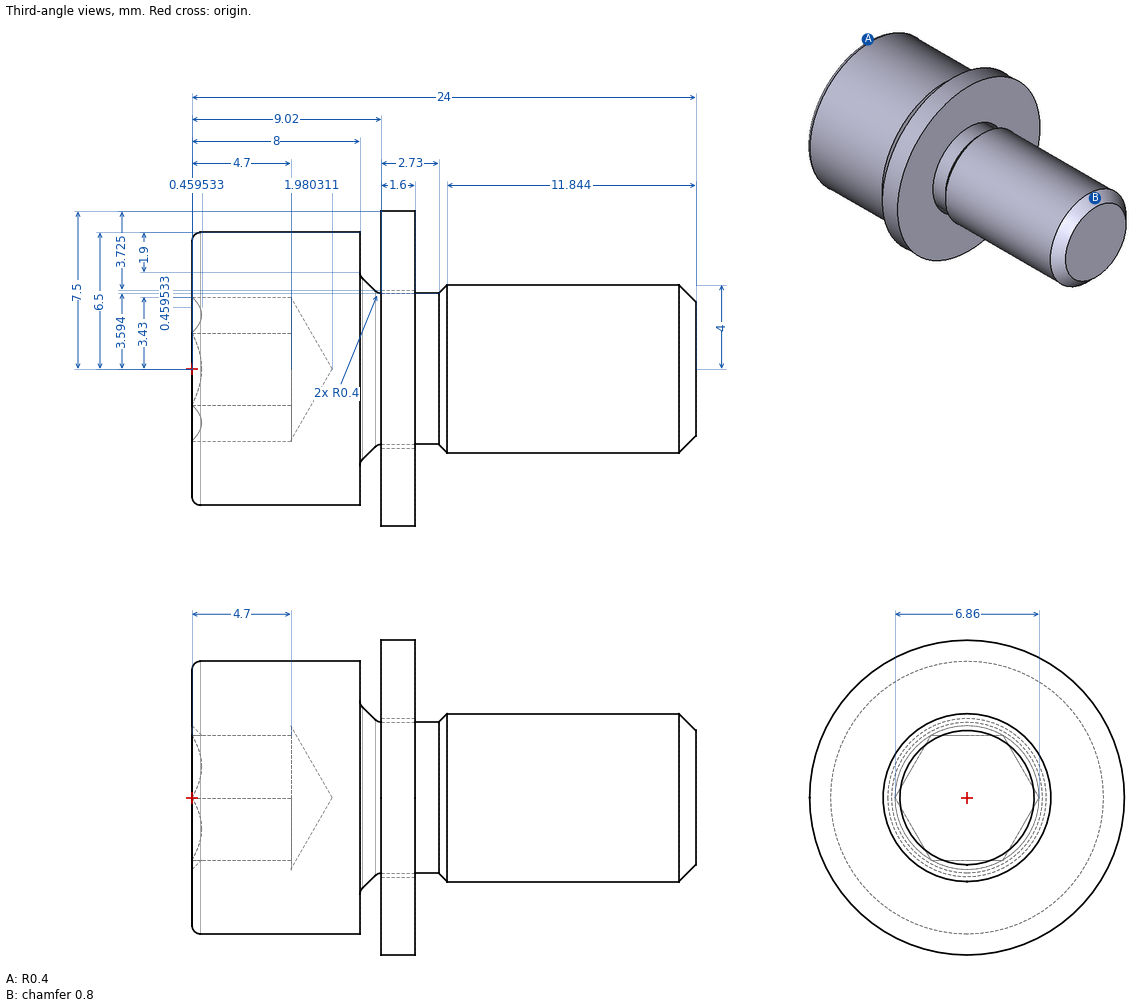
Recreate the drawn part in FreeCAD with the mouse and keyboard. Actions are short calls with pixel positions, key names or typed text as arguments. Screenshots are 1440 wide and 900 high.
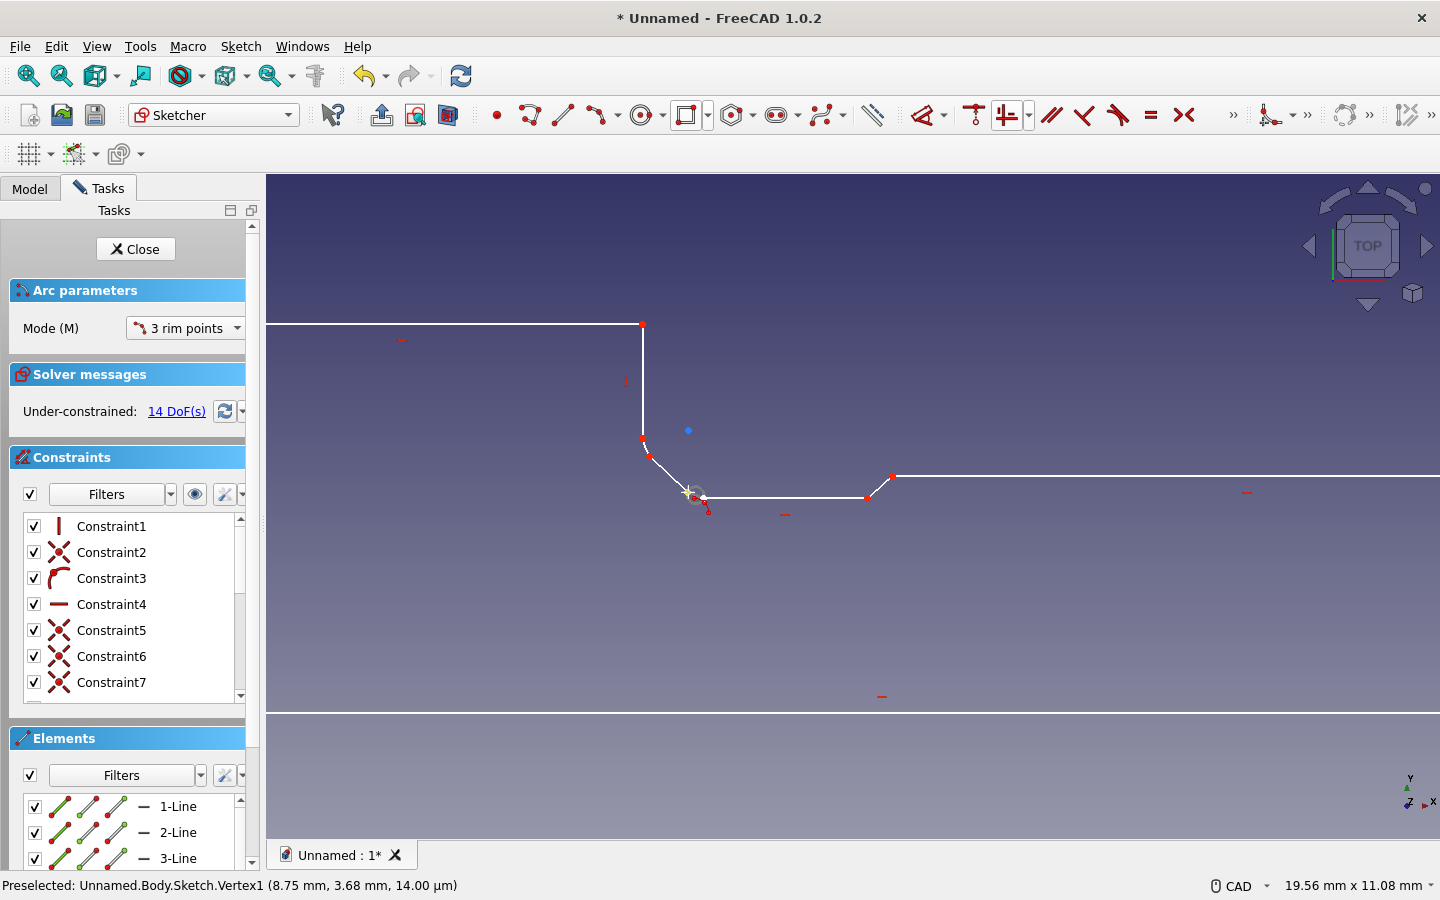
scroll(695, 495, up, 11)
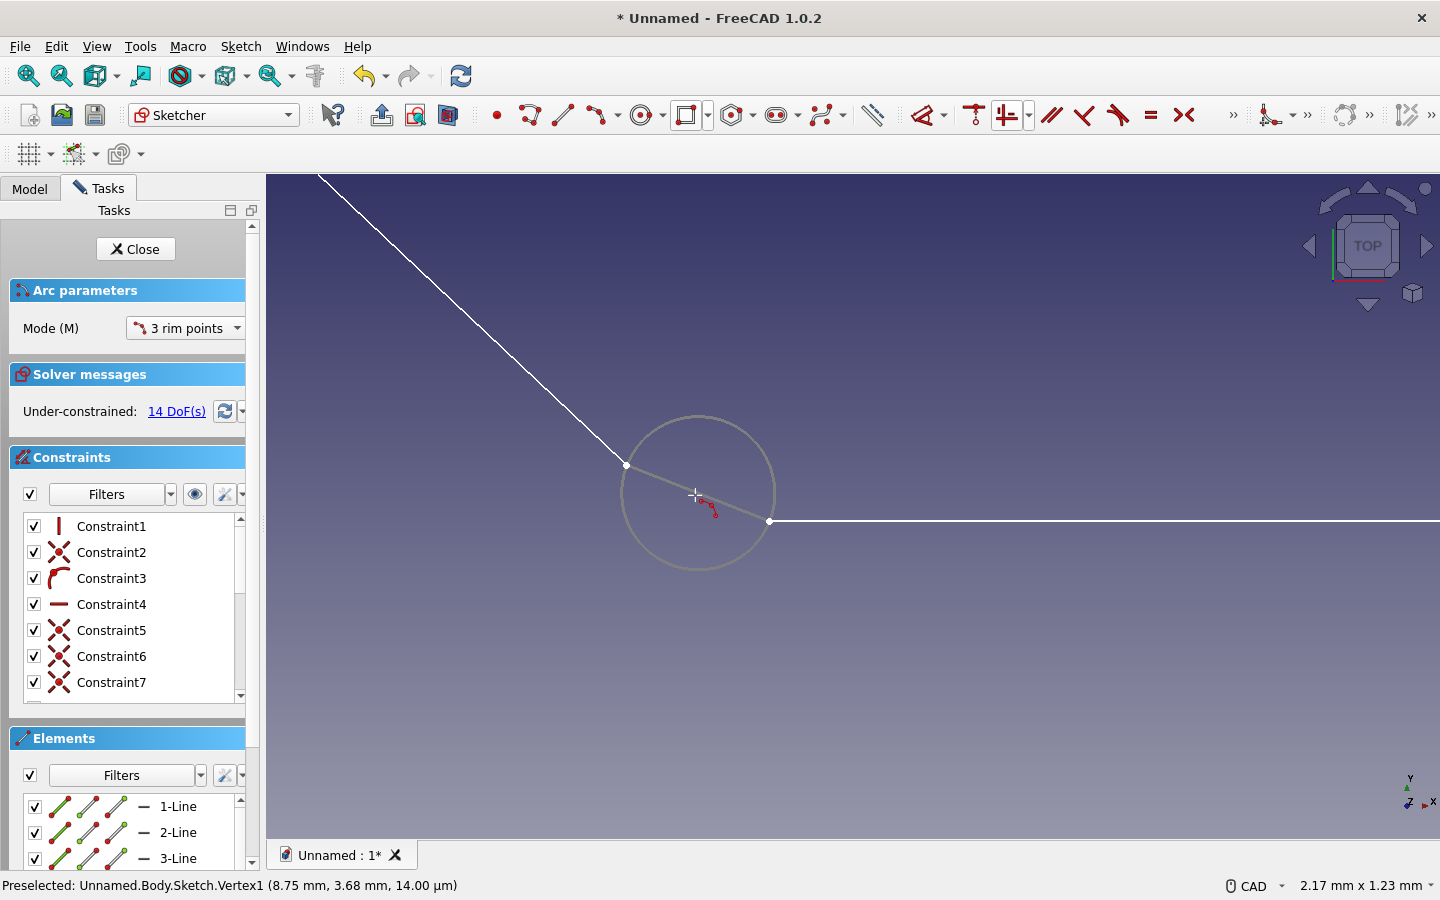
click(692, 494)
key(Escape)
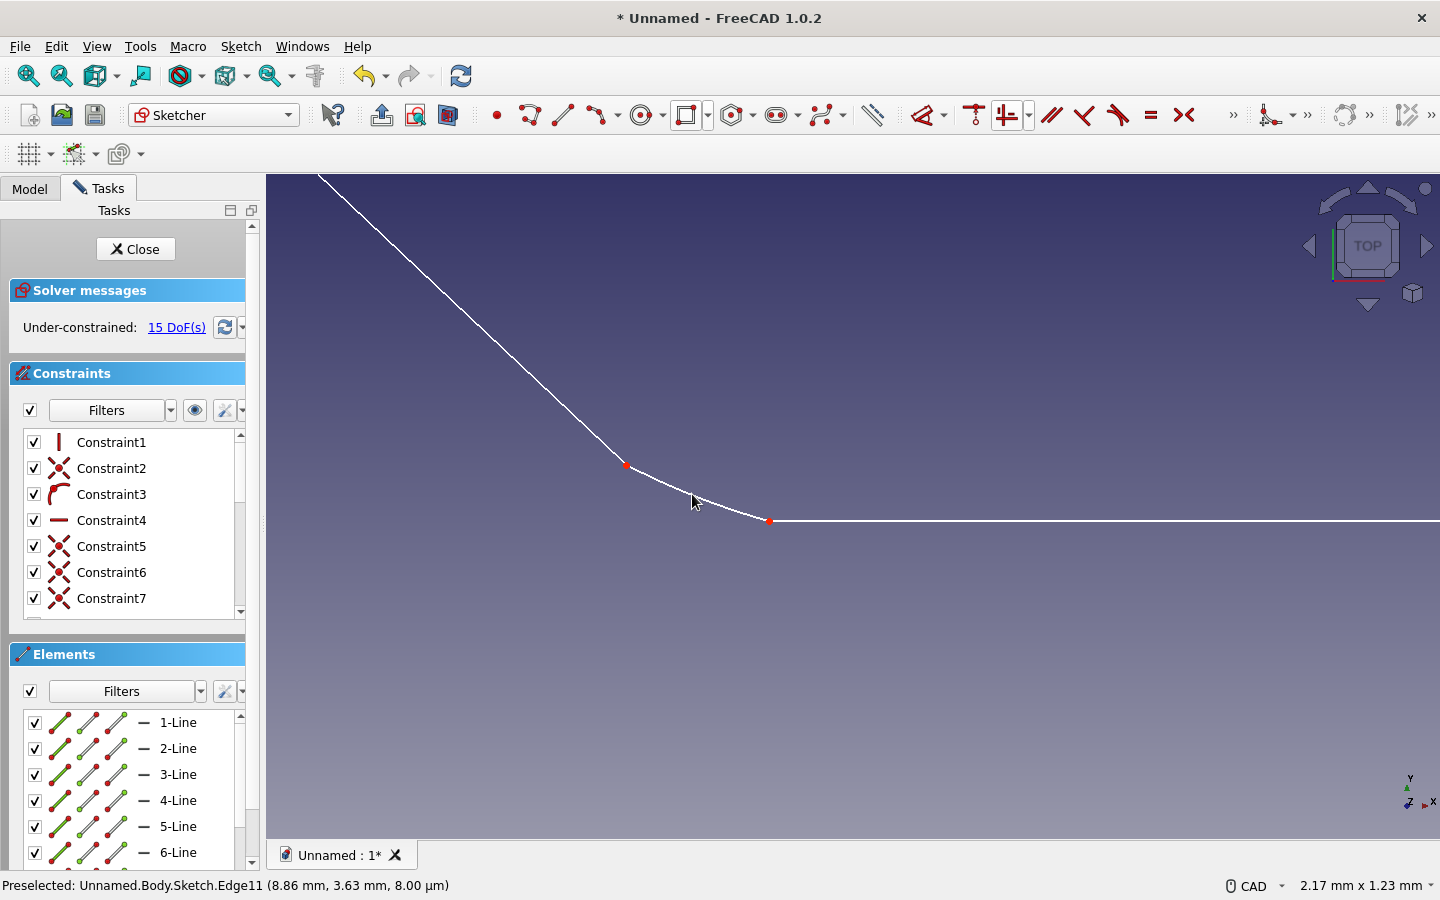
scroll(700, 497, down, 15)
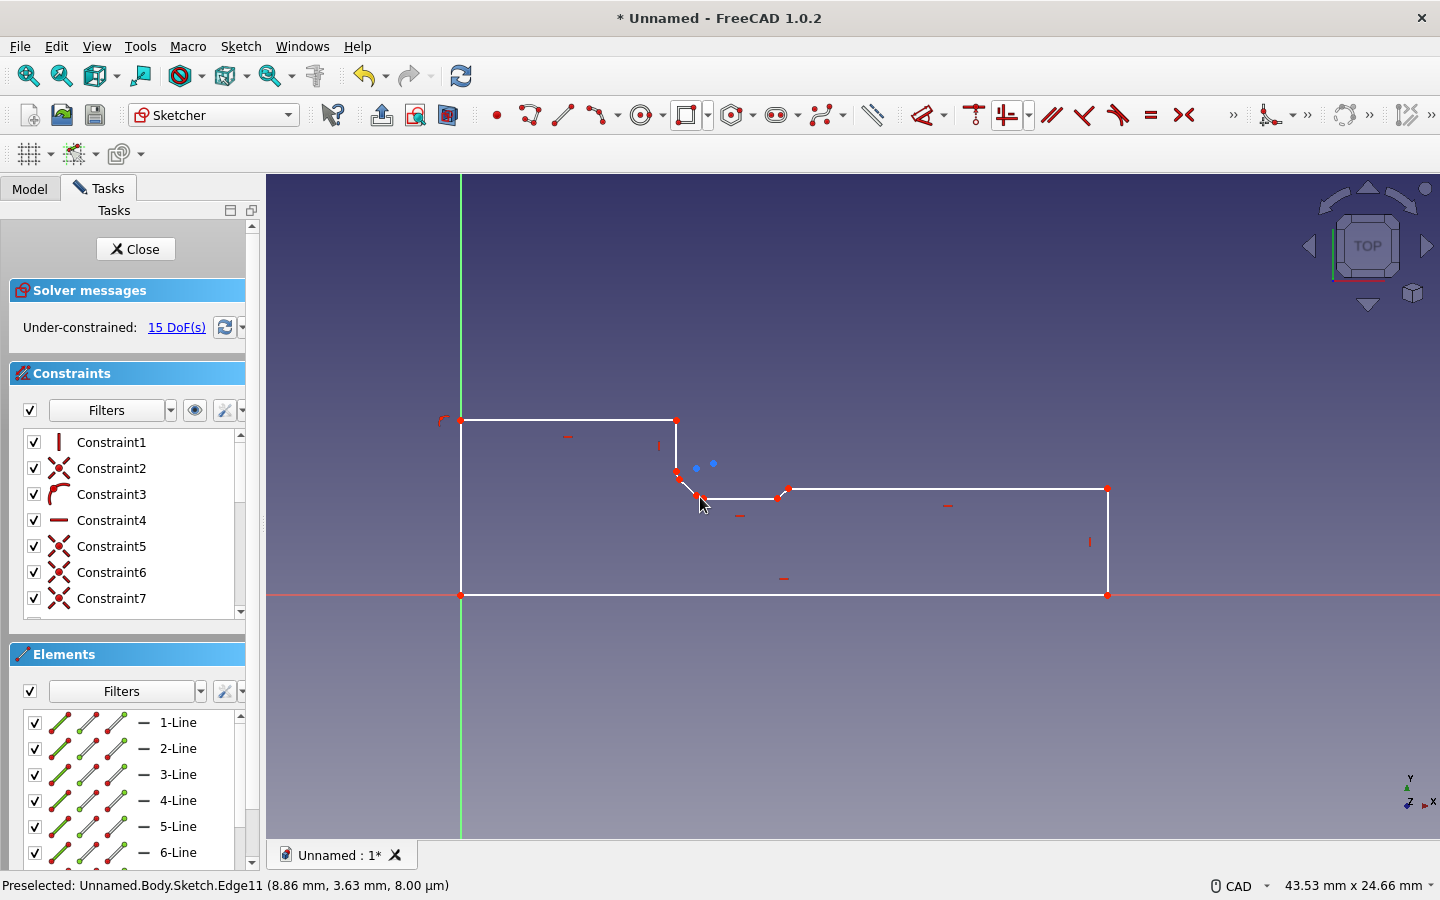
scroll(692, 491, up, 4)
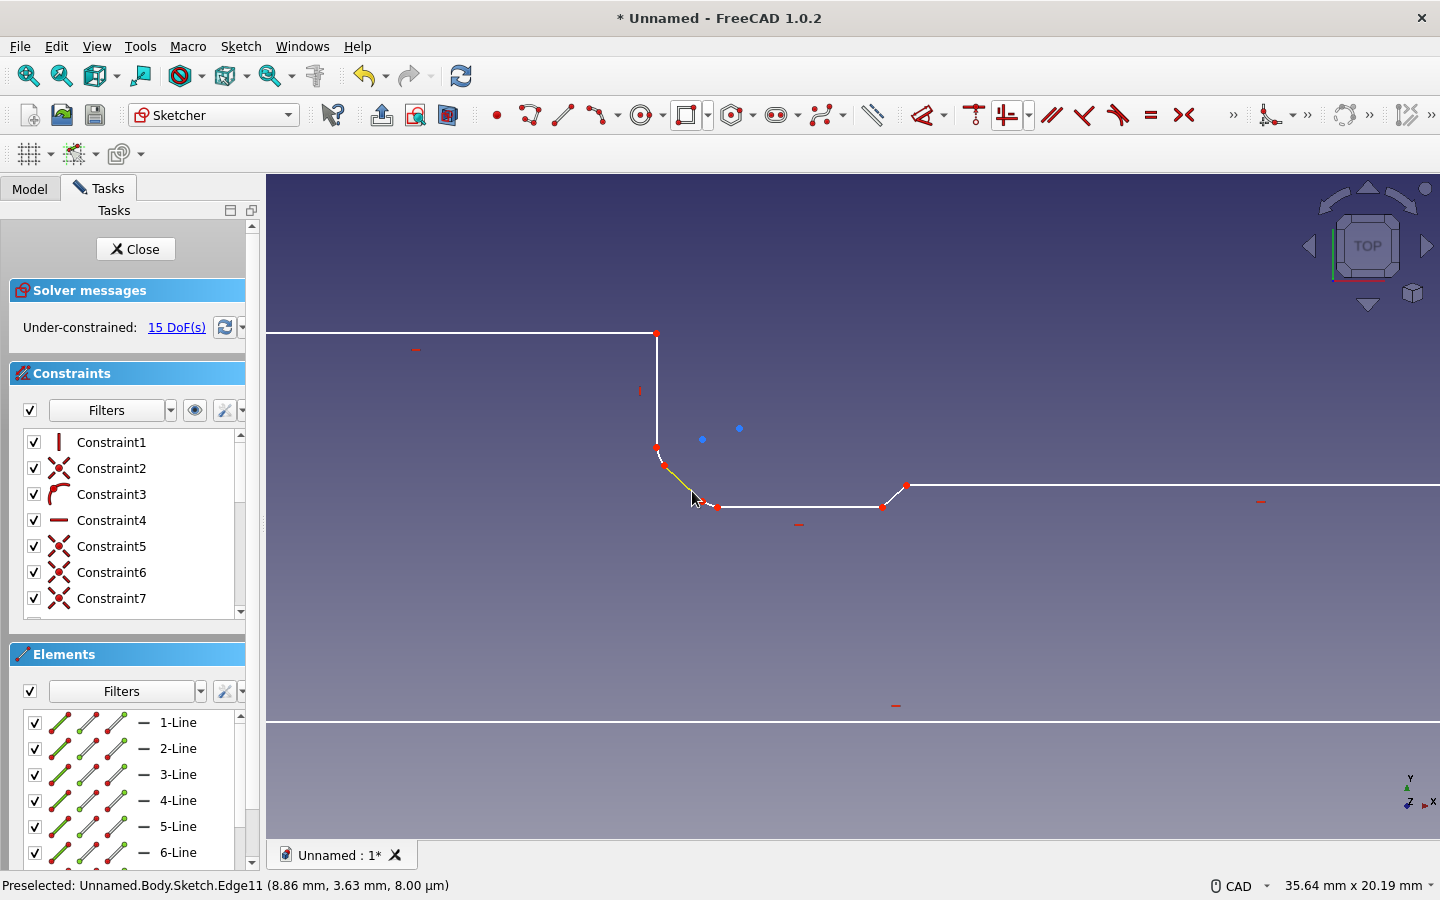
click(691, 491)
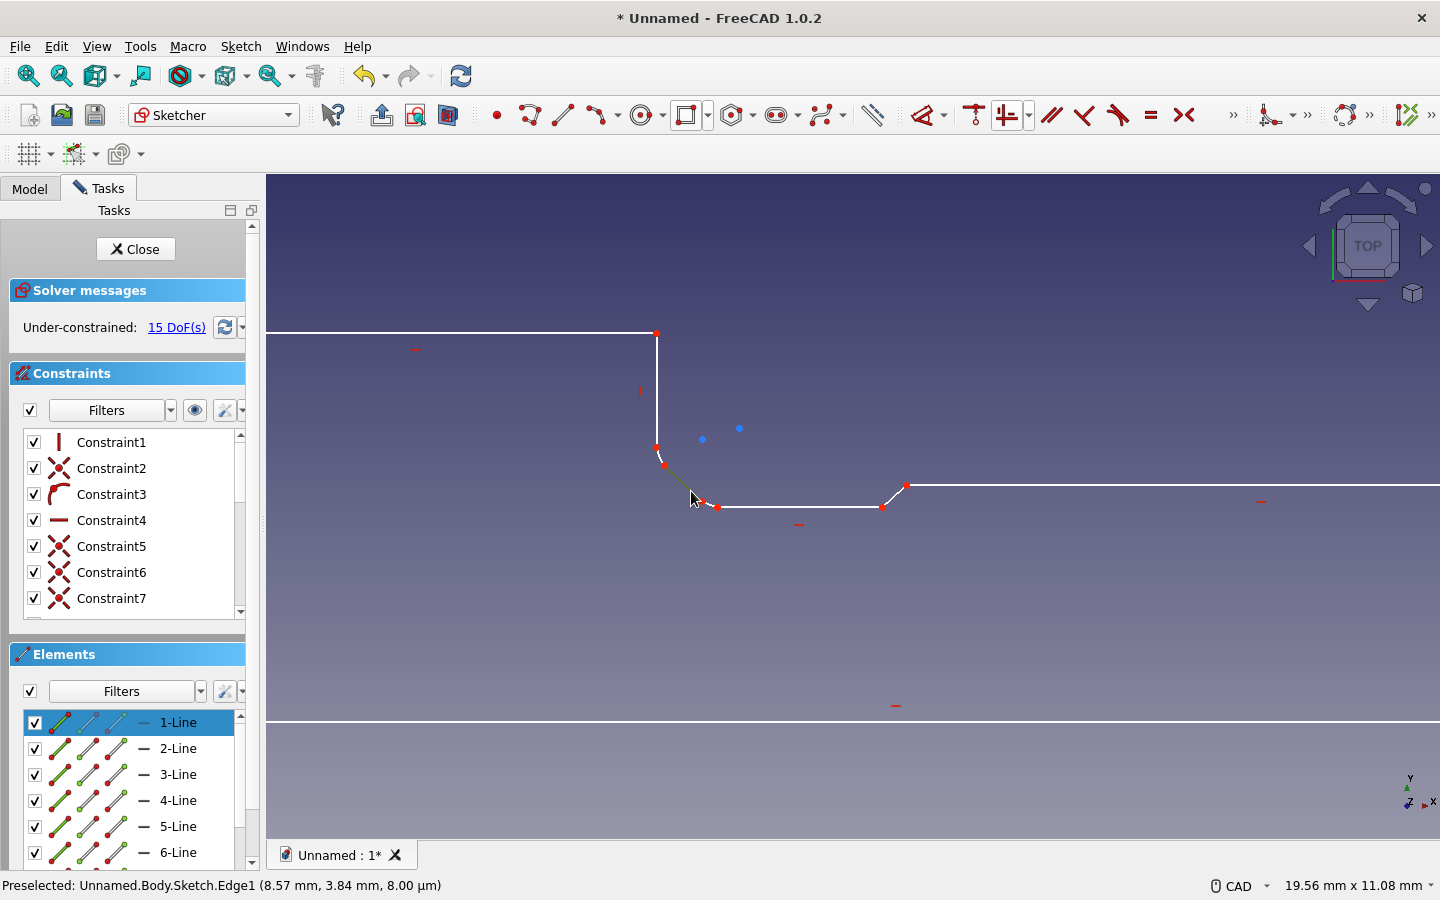
scroll(660, 457, up, 2)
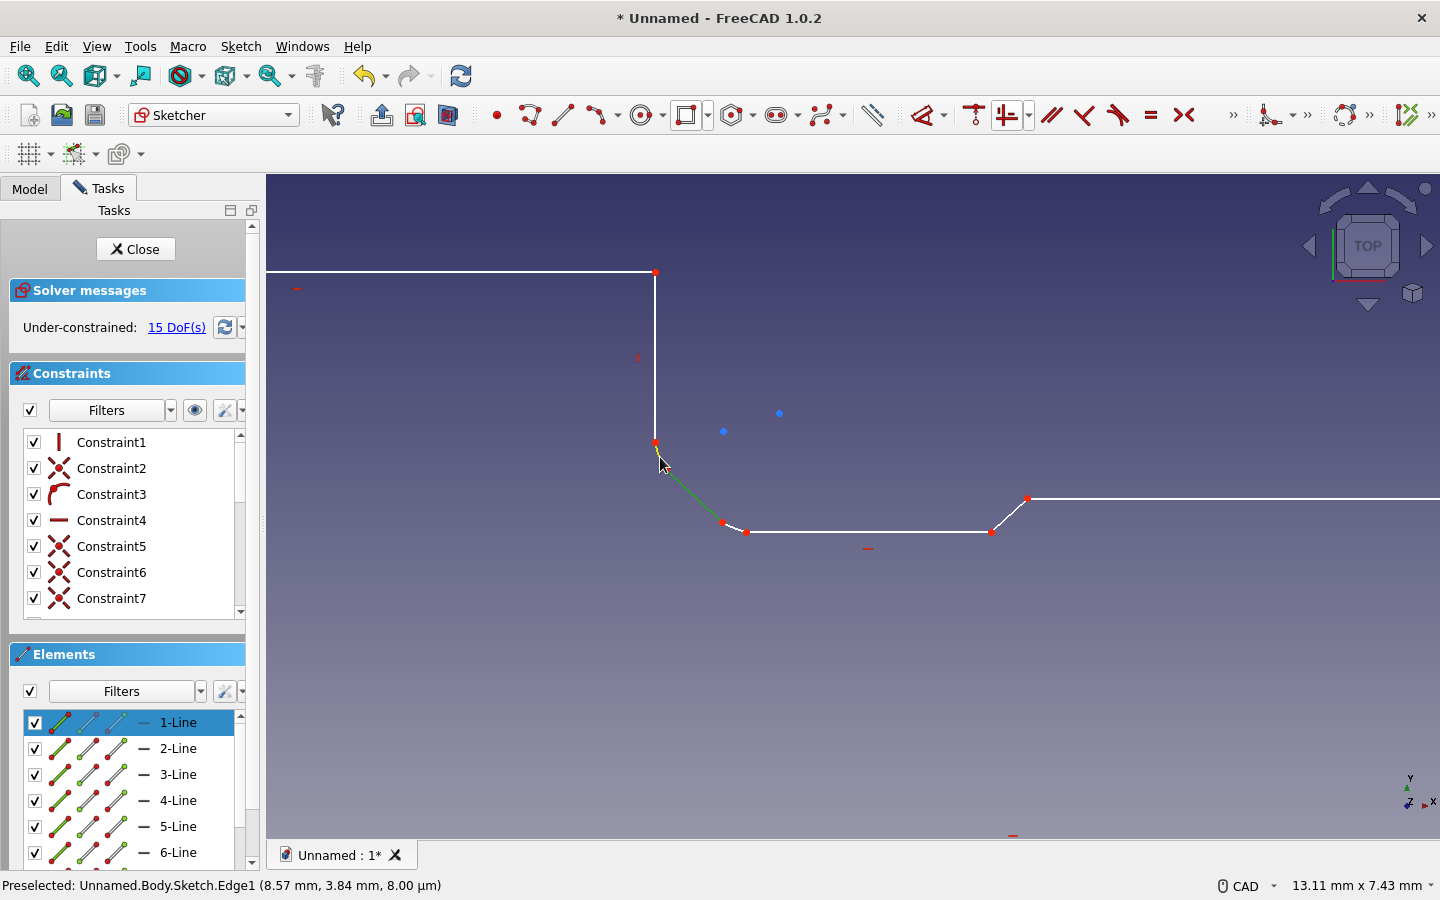
click(659, 457)